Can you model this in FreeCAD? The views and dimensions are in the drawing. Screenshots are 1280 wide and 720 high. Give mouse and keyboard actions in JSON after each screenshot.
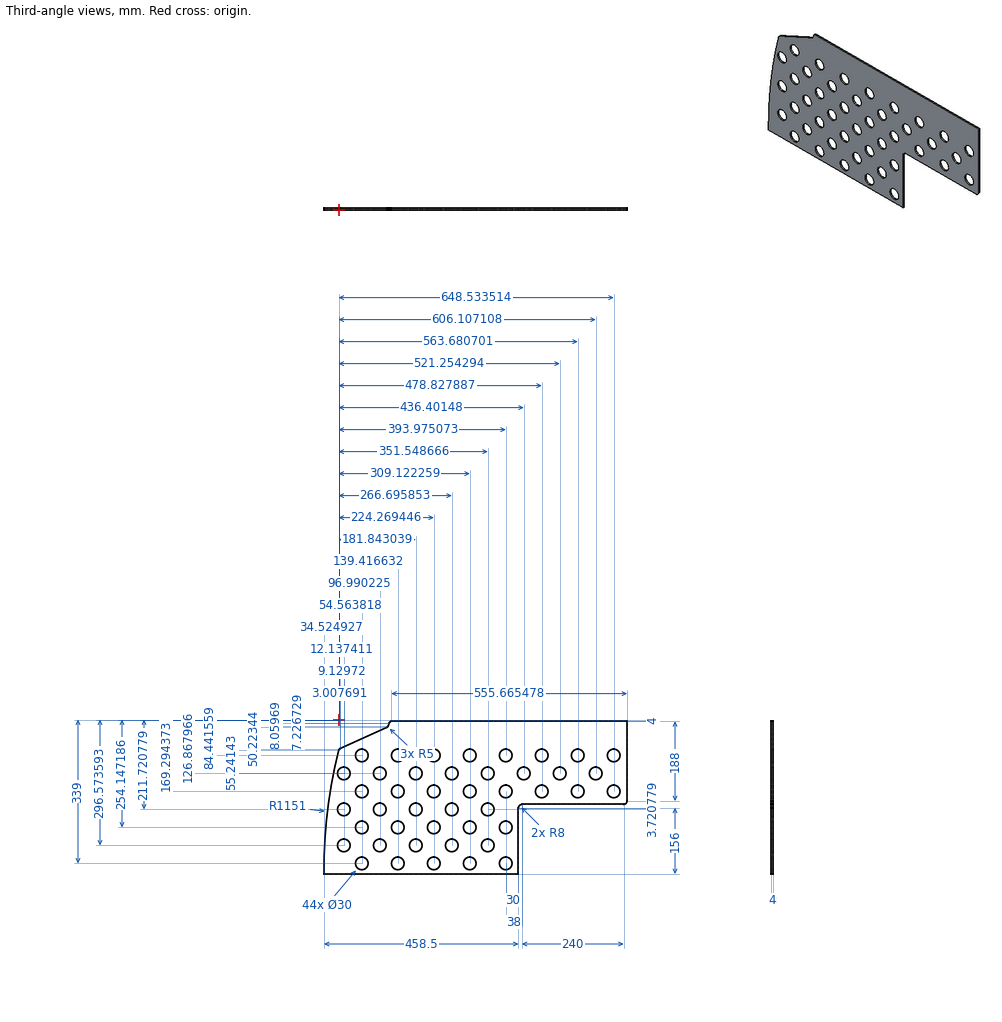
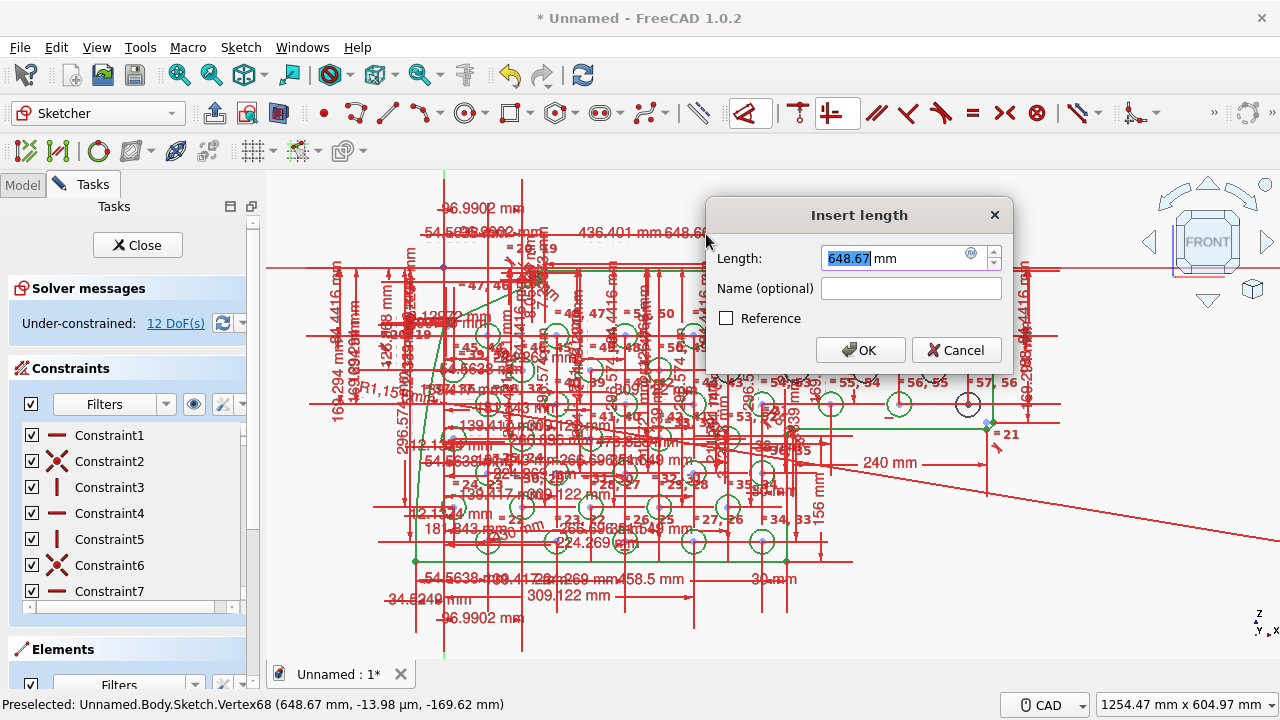
{"action": "type", "text": "648.533514"}
{"action": "key", "text": "Return"}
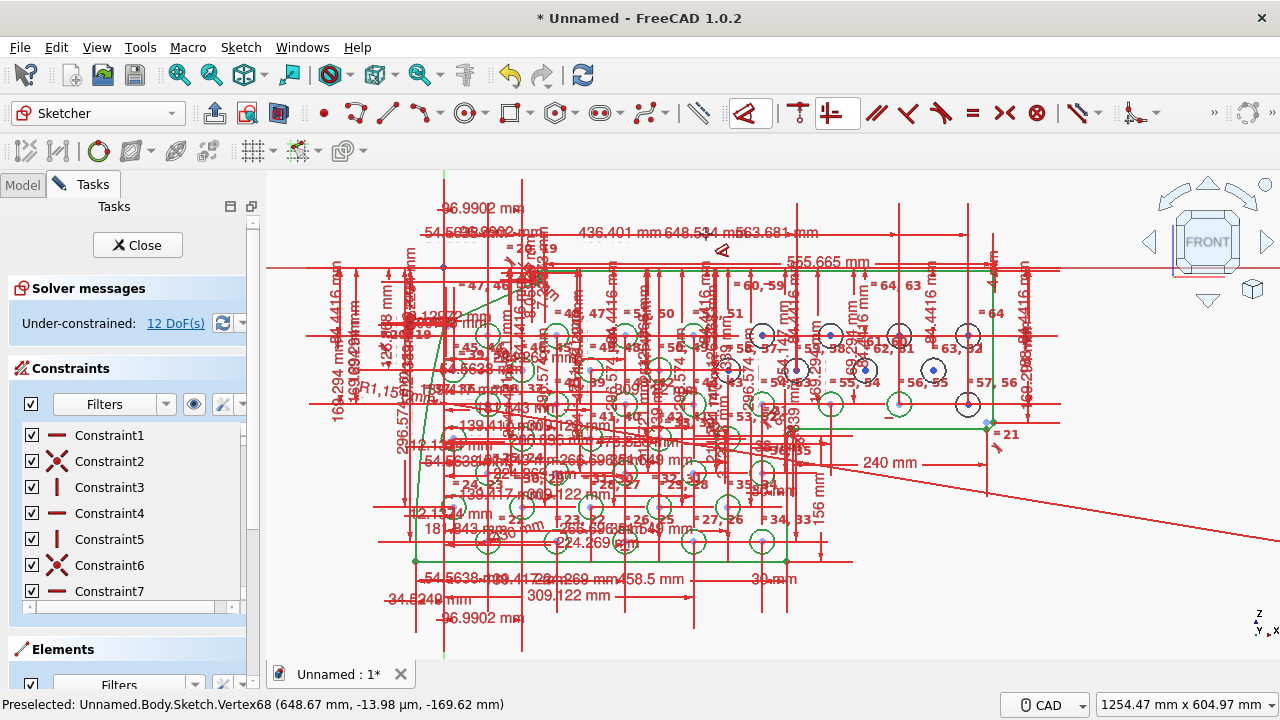
{"action": "left_click", "coordinate": [968, 405]}
{"action": "left_click", "coordinate": [1098, 336]}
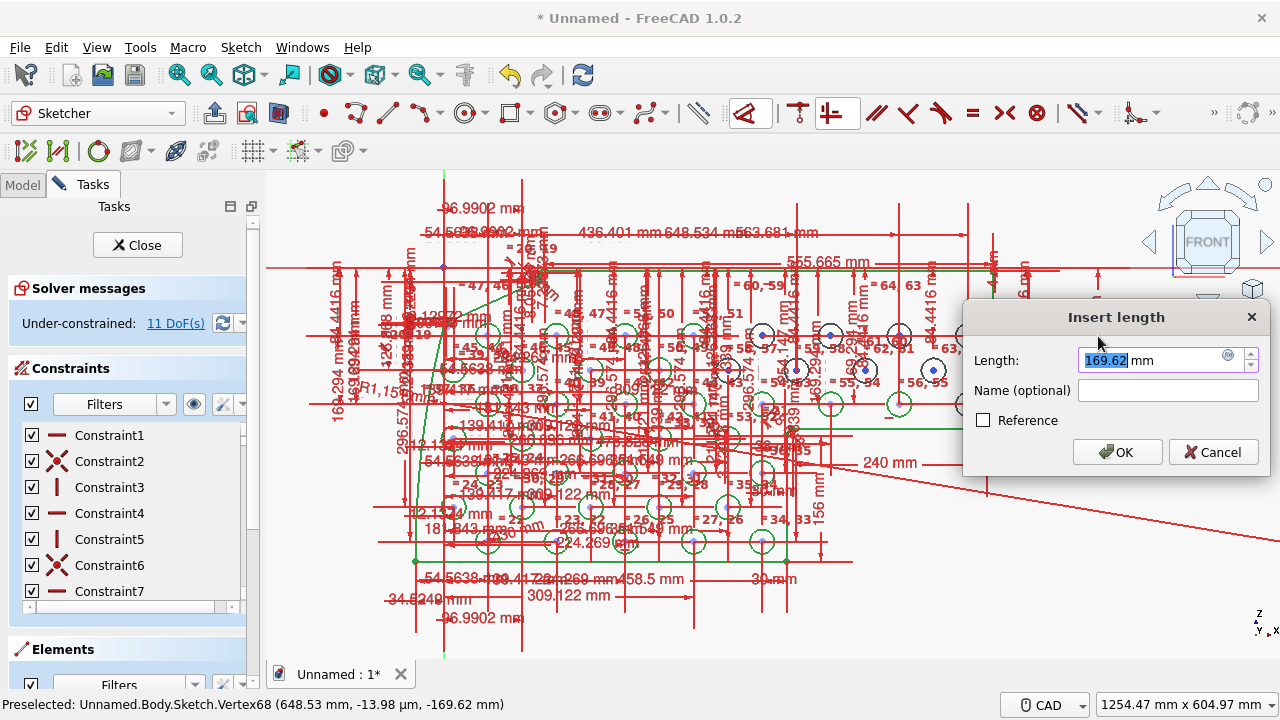
{"action": "type", "text": "169.294373"}
{"action": "key", "text": "Return"}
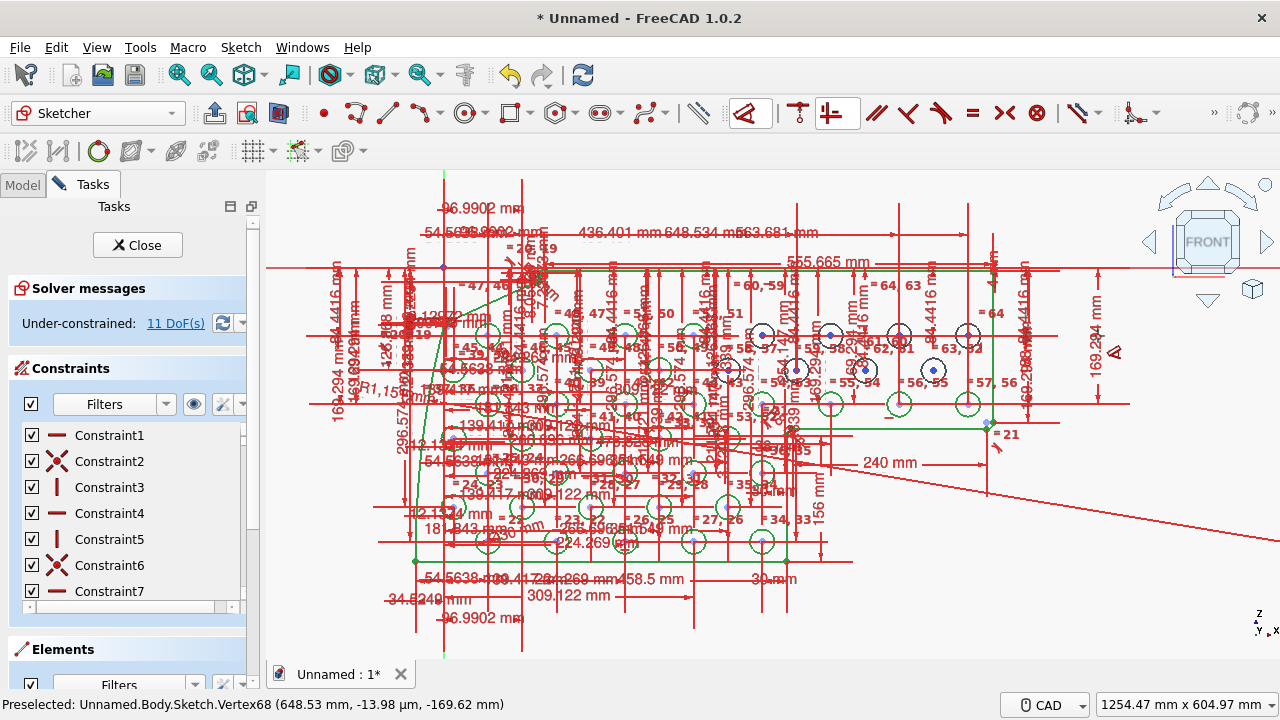
{"action": "left_click", "coordinate": [728, 371]}
{"action": "left_click", "coordinate": [586, 210]}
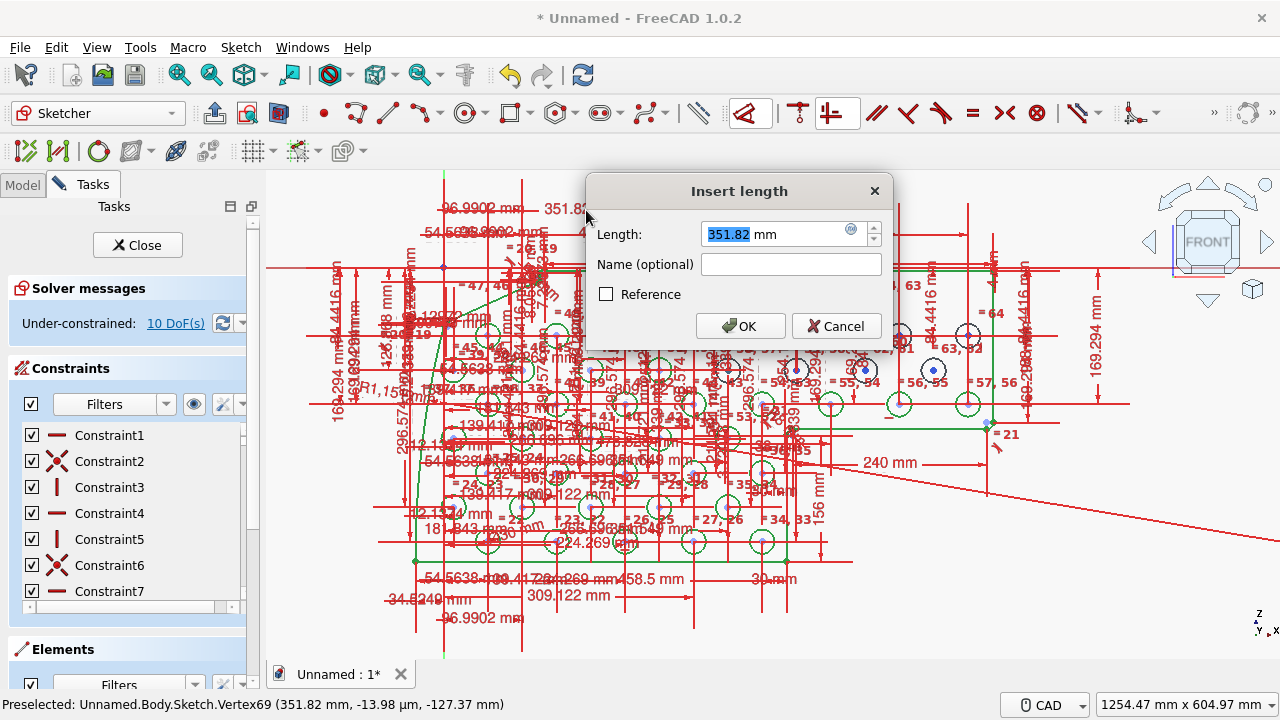
{"action": "type", "text": "351.548666"}
{"action": "key", "text": "Return"}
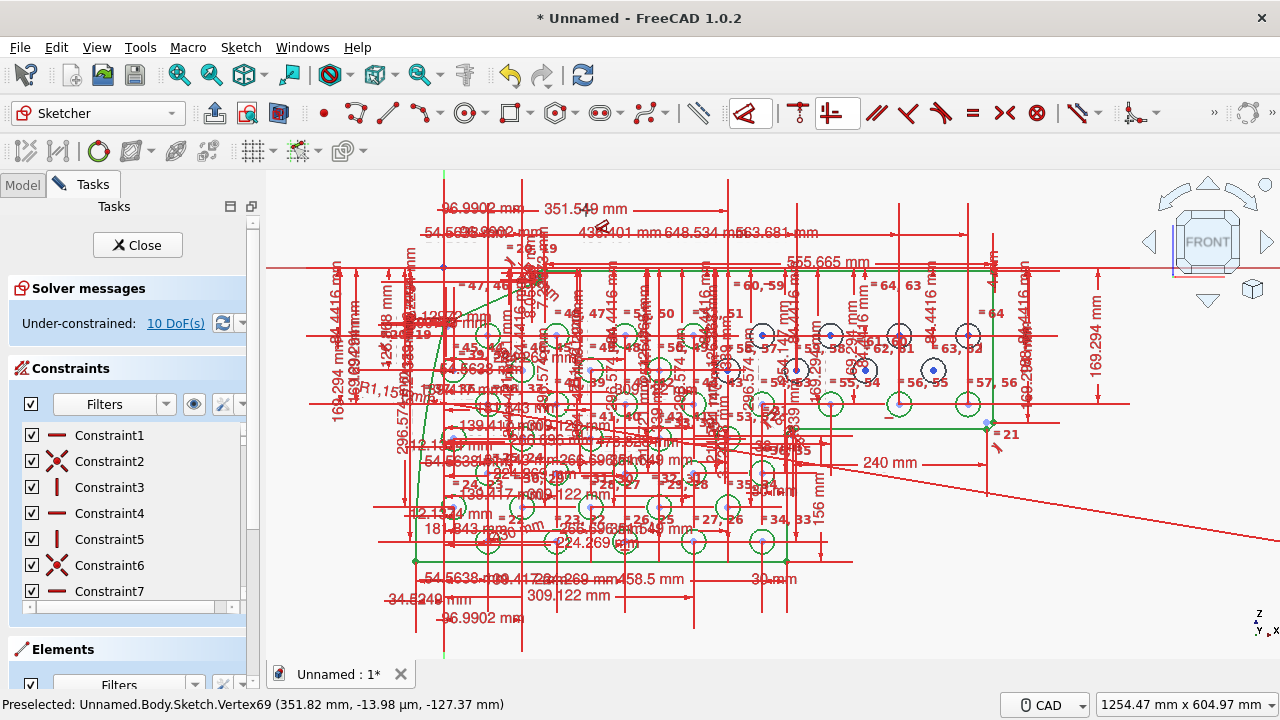
{"action": "left_click", "coordinate": [728, 371]}
{"action": "left_click", "coordinate": [762, 283]}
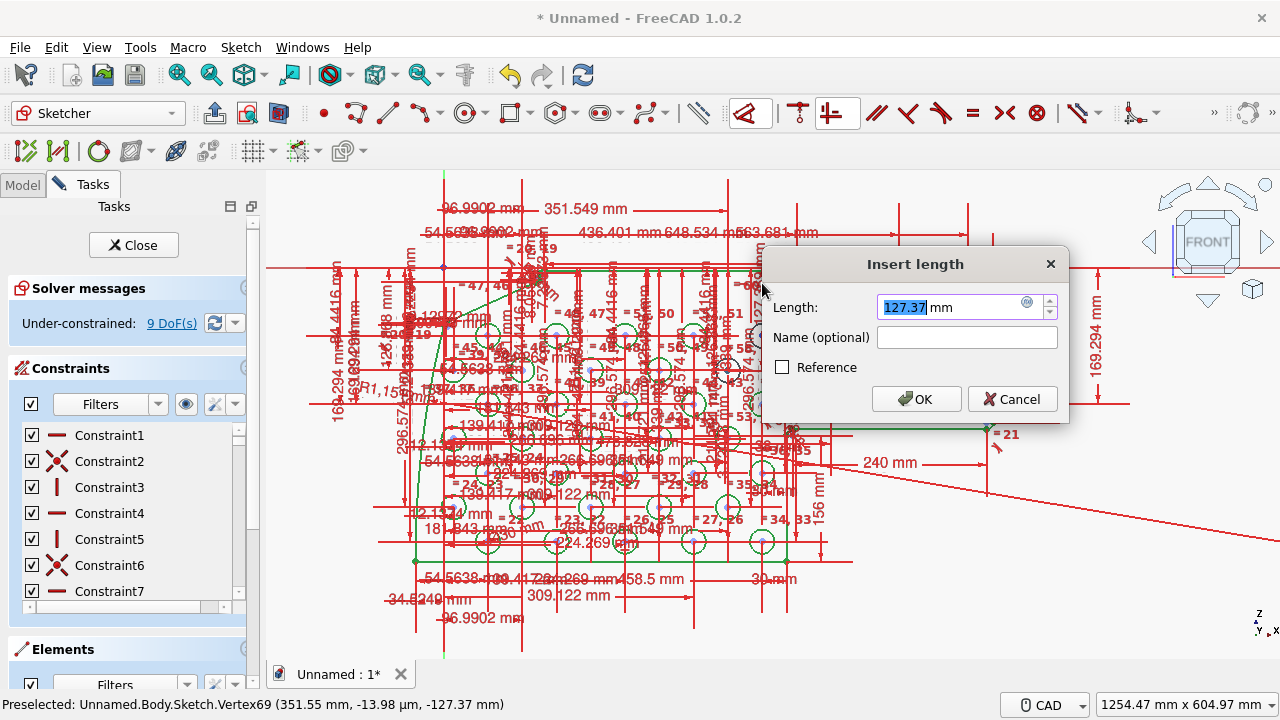
{"action": "type", "text": "126.867966"}
{"action": "key", "text": "Return"}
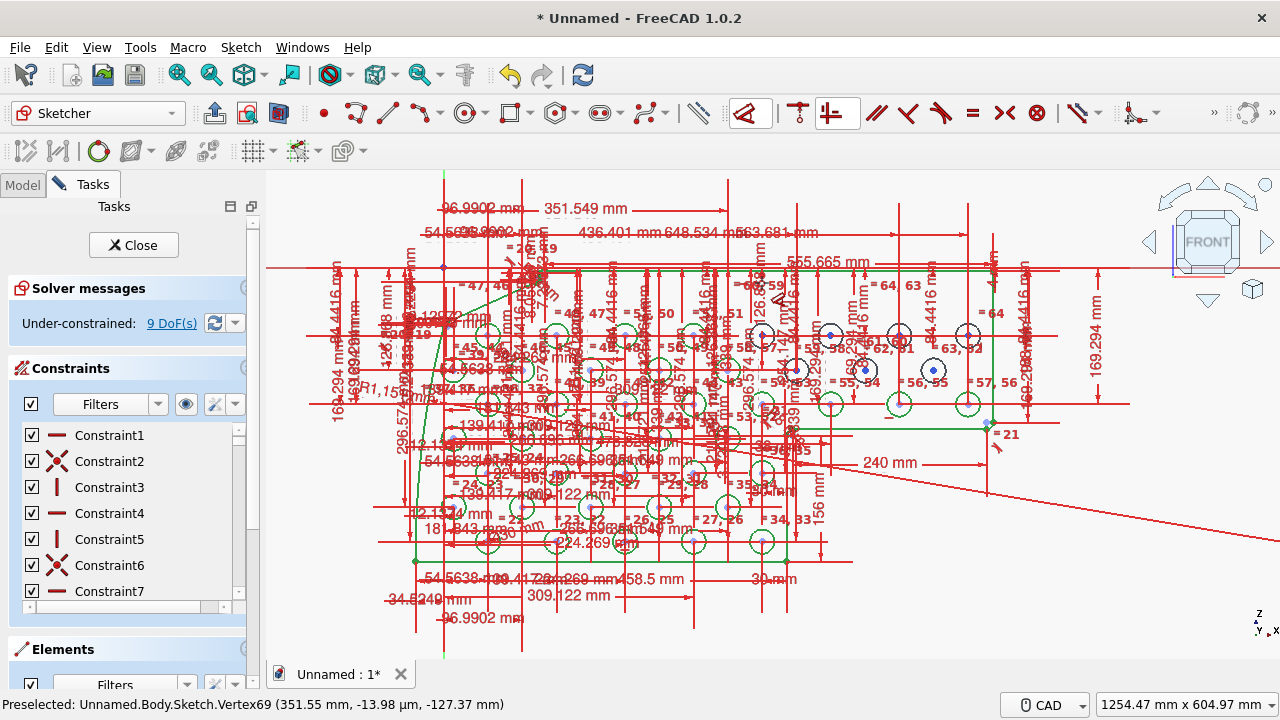
{"action": "left_click", "coordinate": [797, 371]}
{"action": "left_click", "coordinate": [831, 283]}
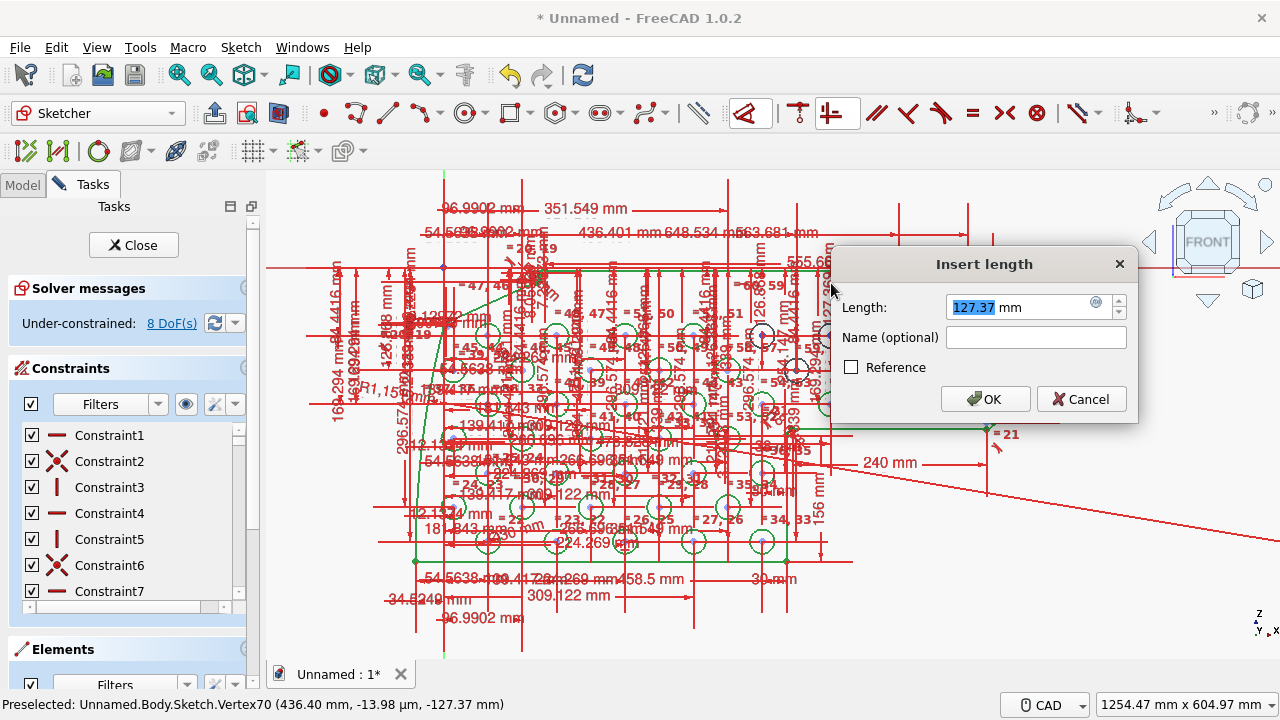
{"action": "type", "text": "126.867966"}
{"action": "key", "text": "Return"}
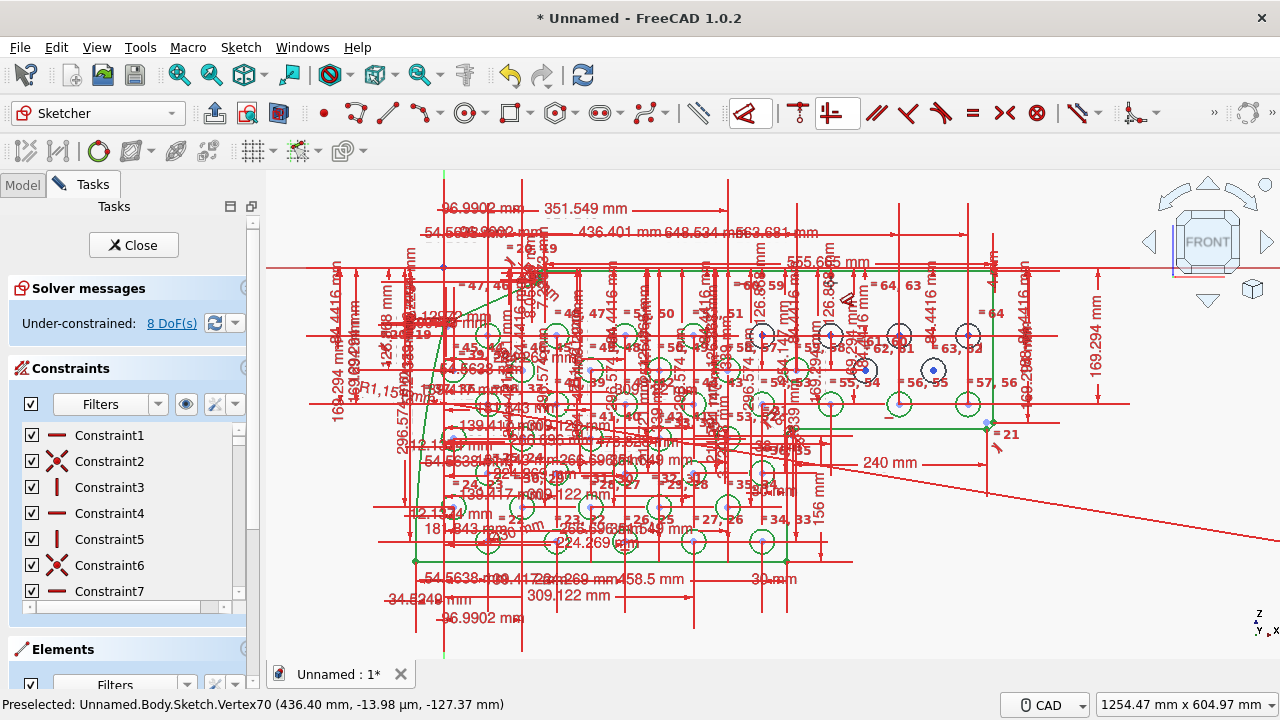
{"action": "left_click", "coordinate": [762, 336]}
{"action": "left_click", "coordinate": [676, 210]}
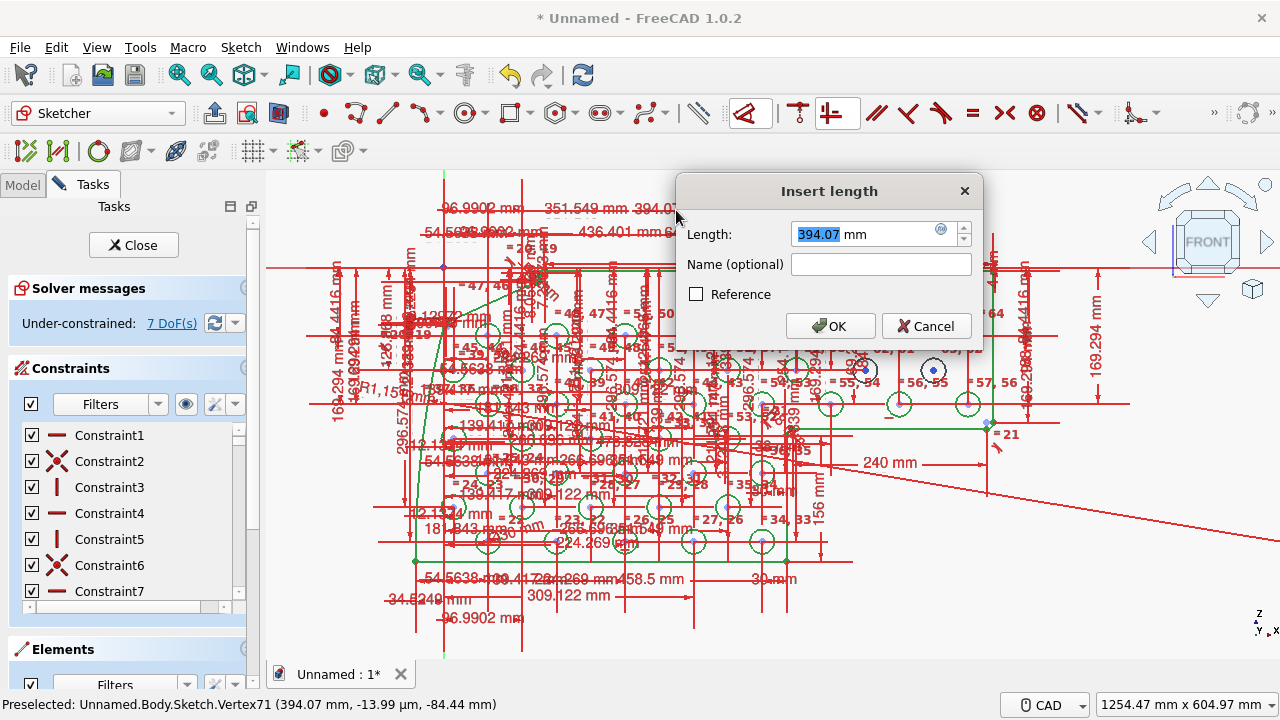
{"action": "type", "text": "393.975073"}
{"action": "key", "text": "Return"}